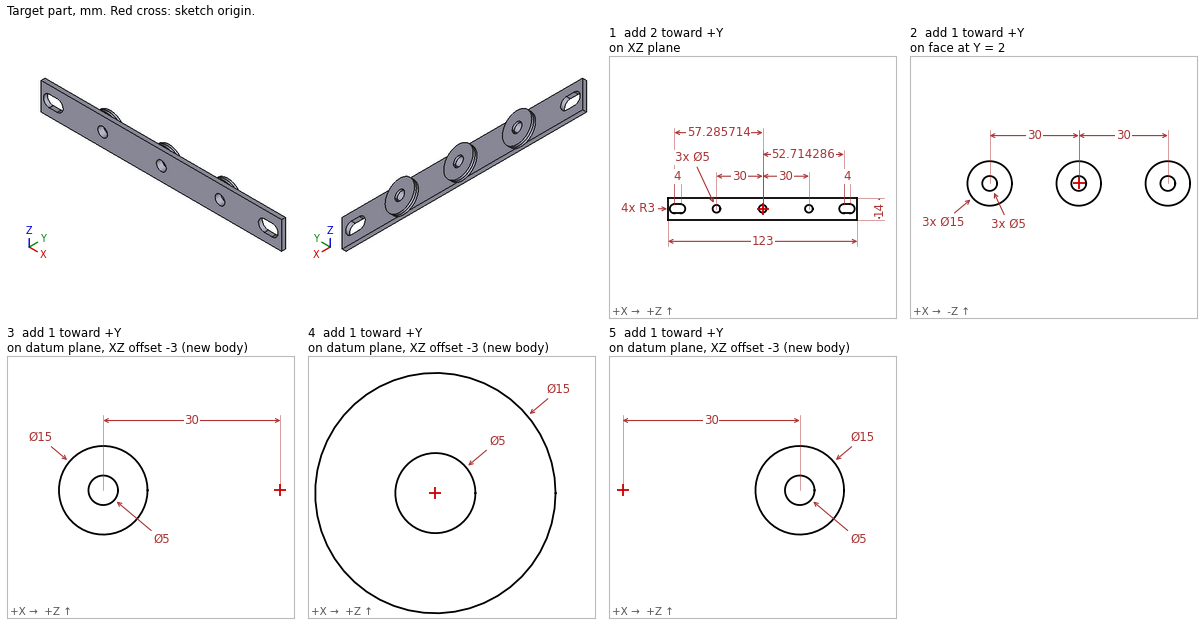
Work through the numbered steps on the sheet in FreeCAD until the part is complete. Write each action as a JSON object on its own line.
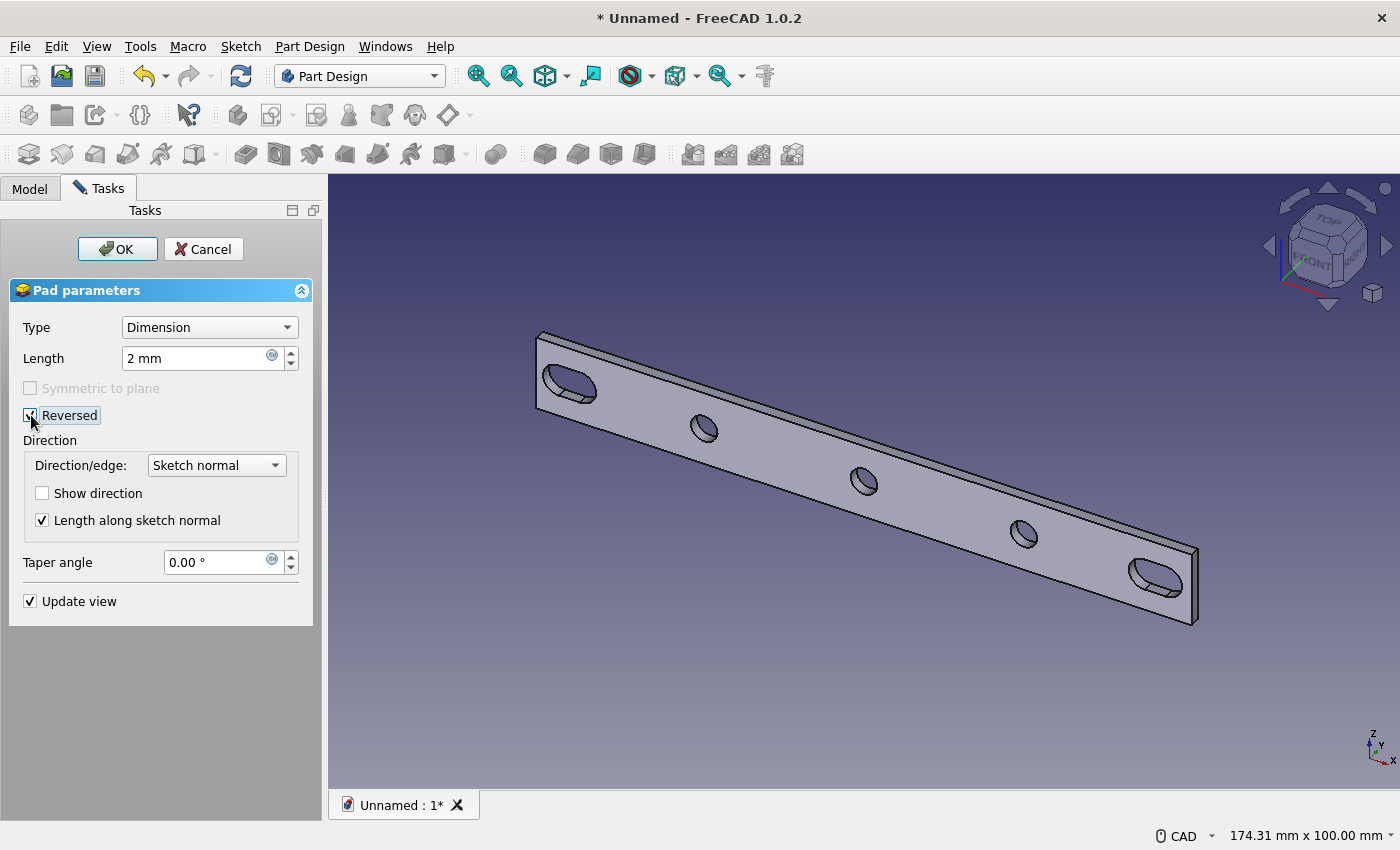
{"action": "left_click", "coordinate": [118, 249]}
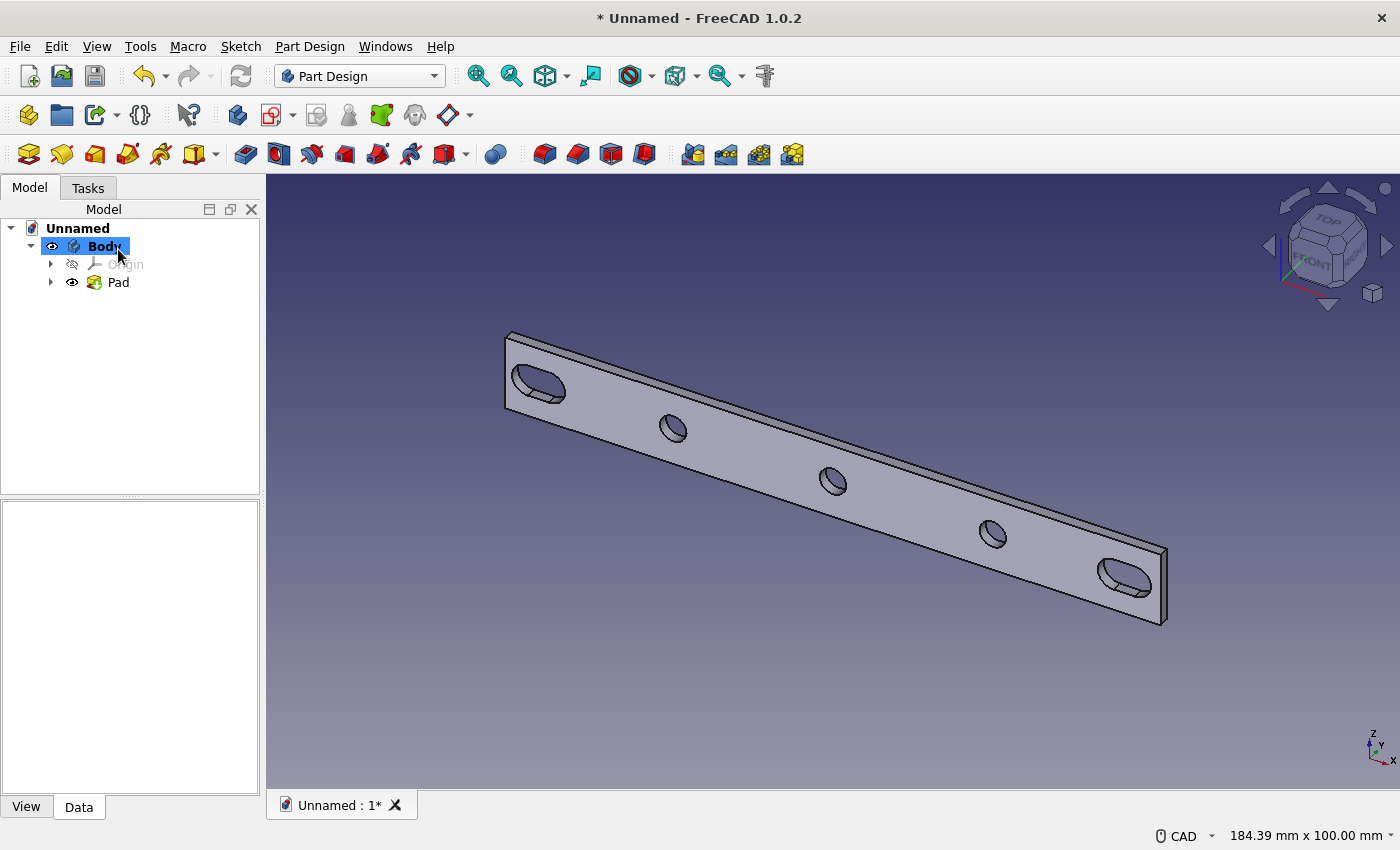
{"action": "key", "text": "4"}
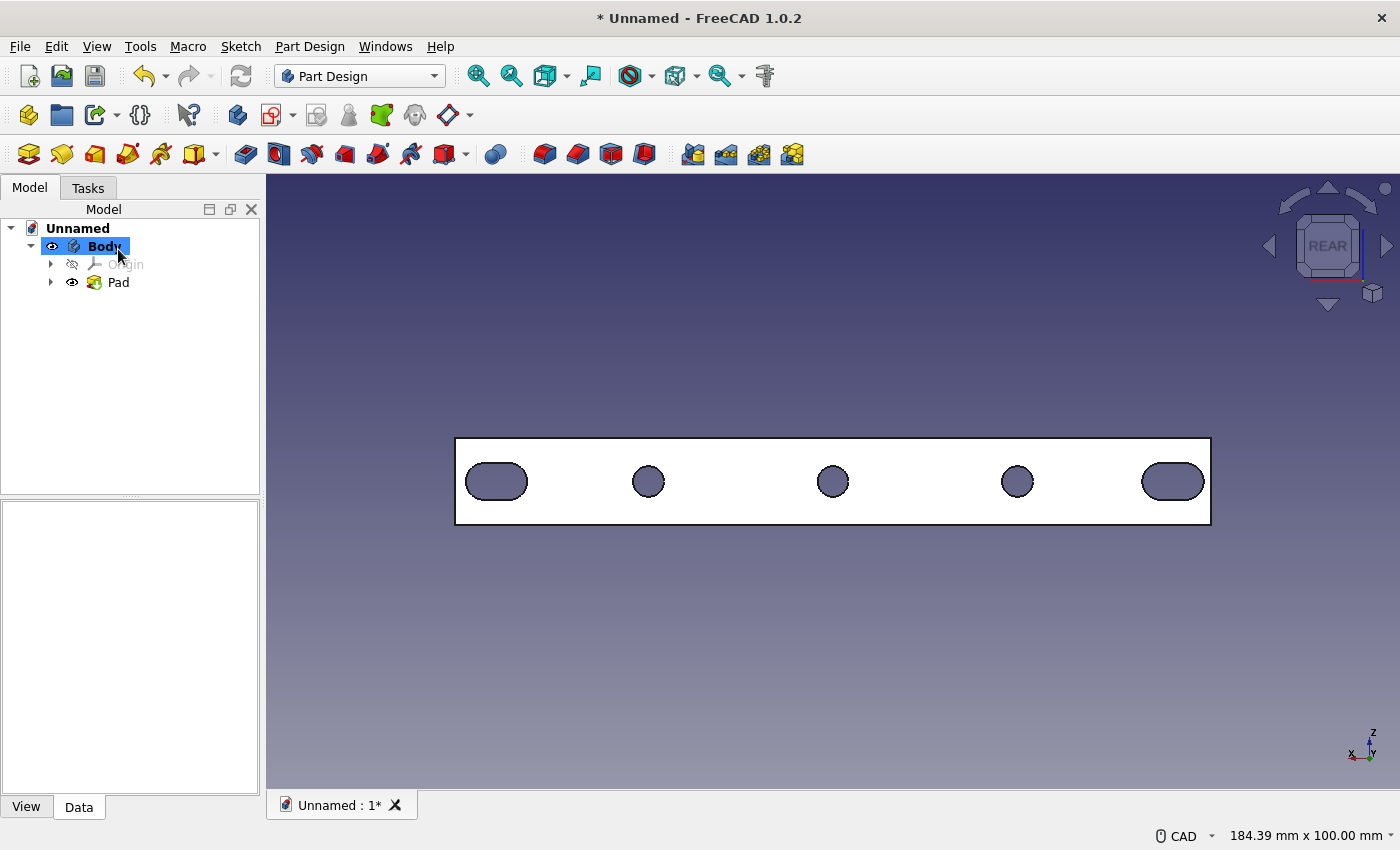
{"action": "left_click", "coordinate": [725, 480]}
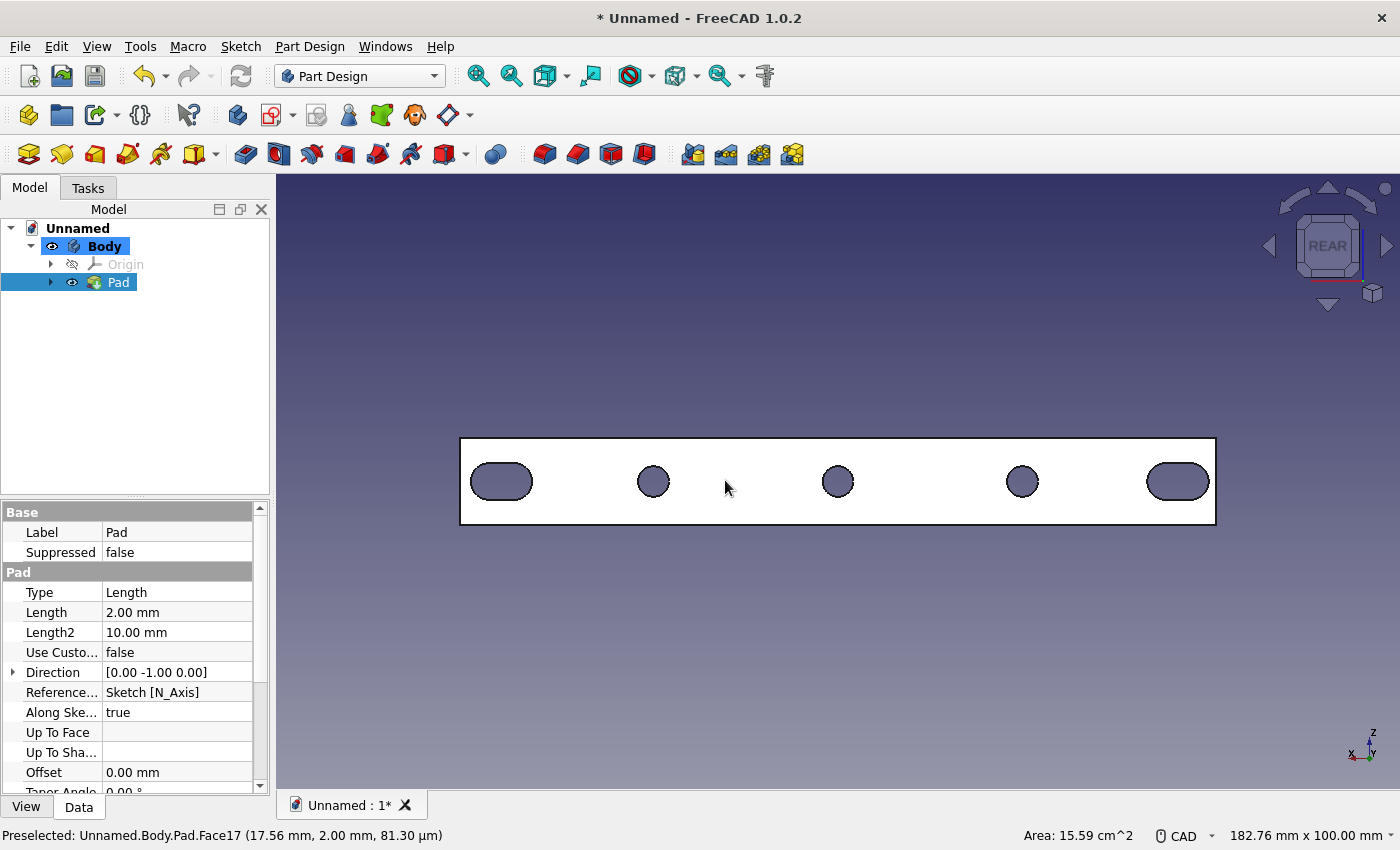
{"action": "left_click", "coordinate": [270, 116]}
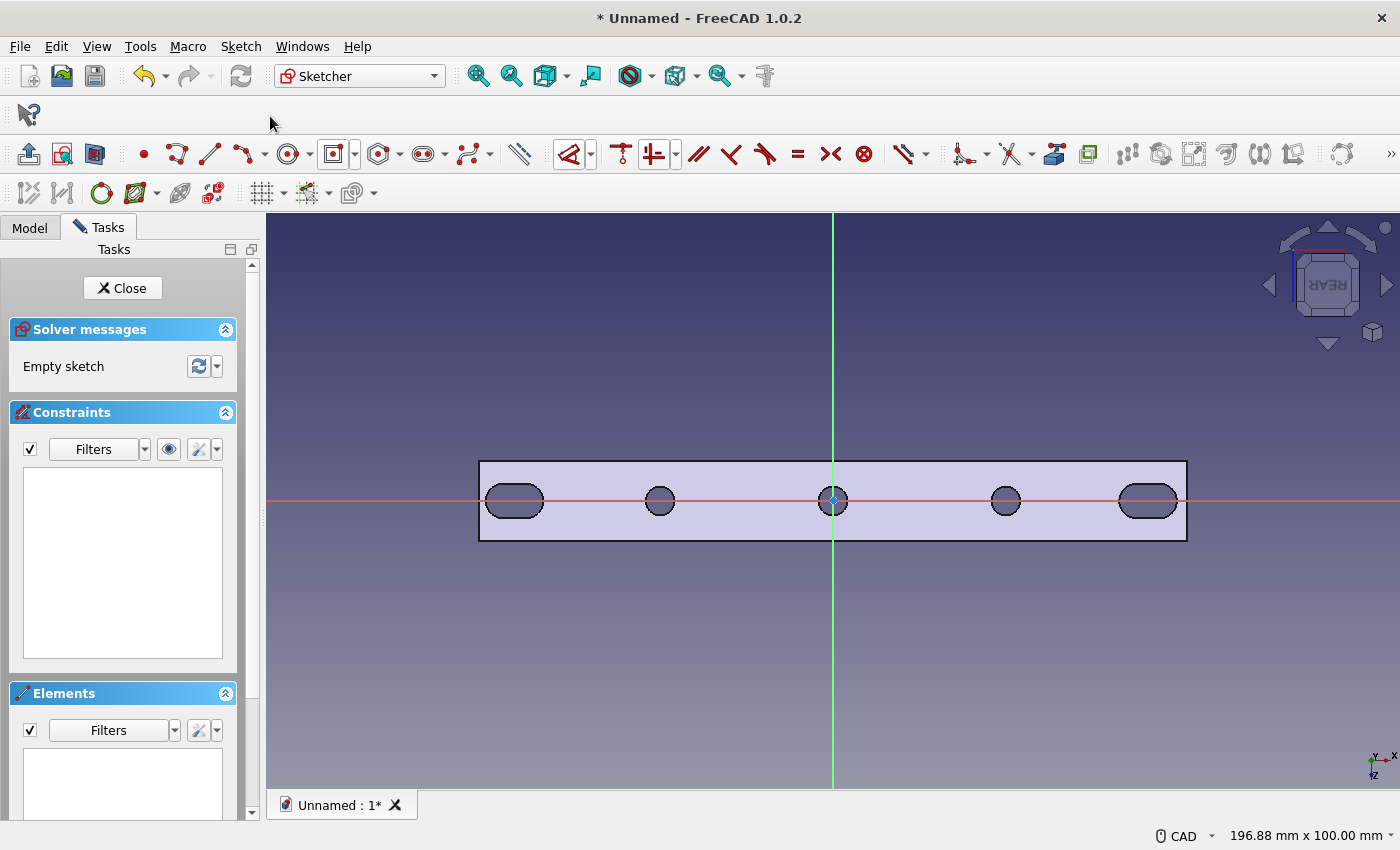
{"action": "scroll", "coordinate": [972, 501], "scroll_direction": "up", "scroll_amount": 2}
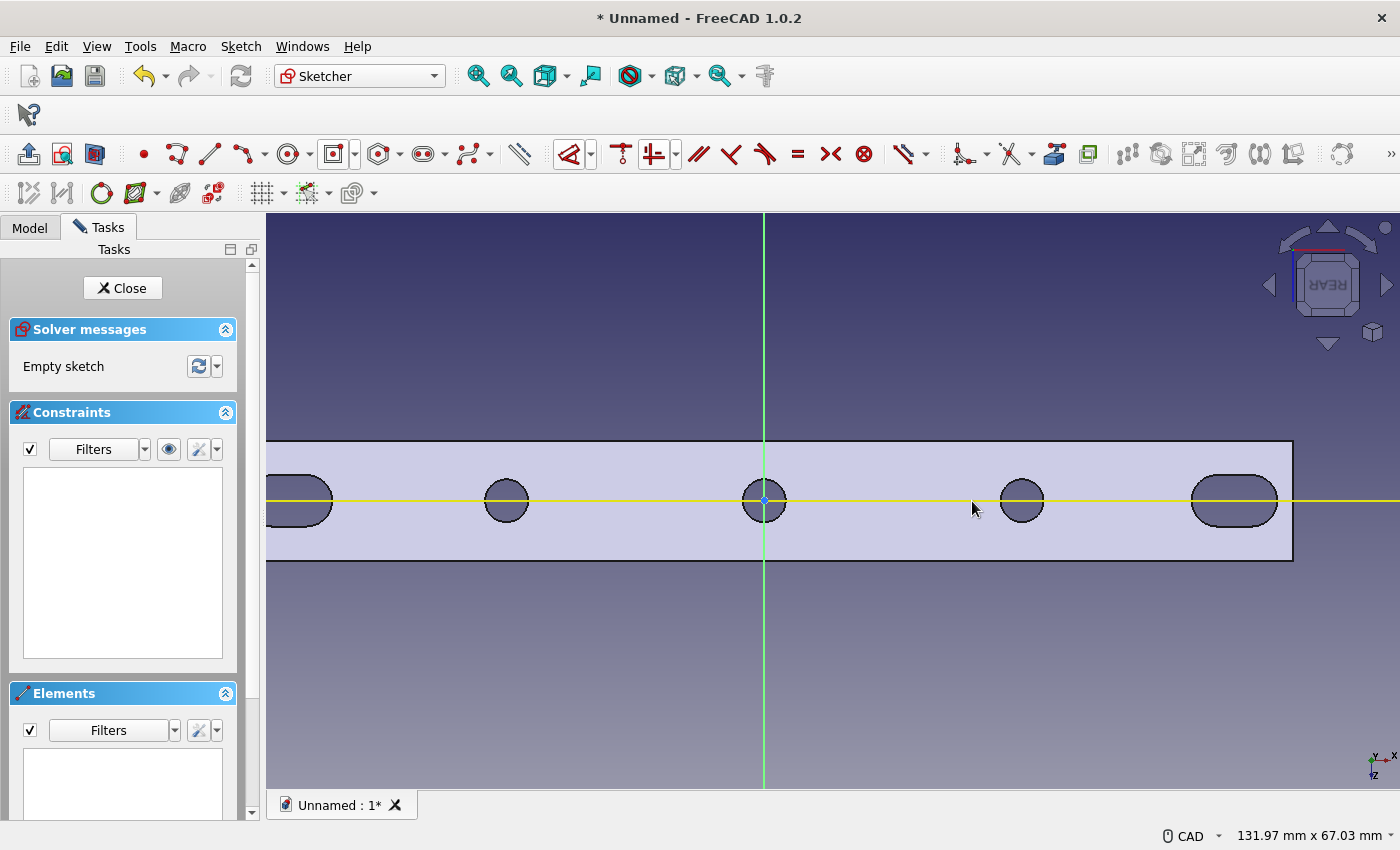
{"action": "left_click", "coordinate": [288, 154]}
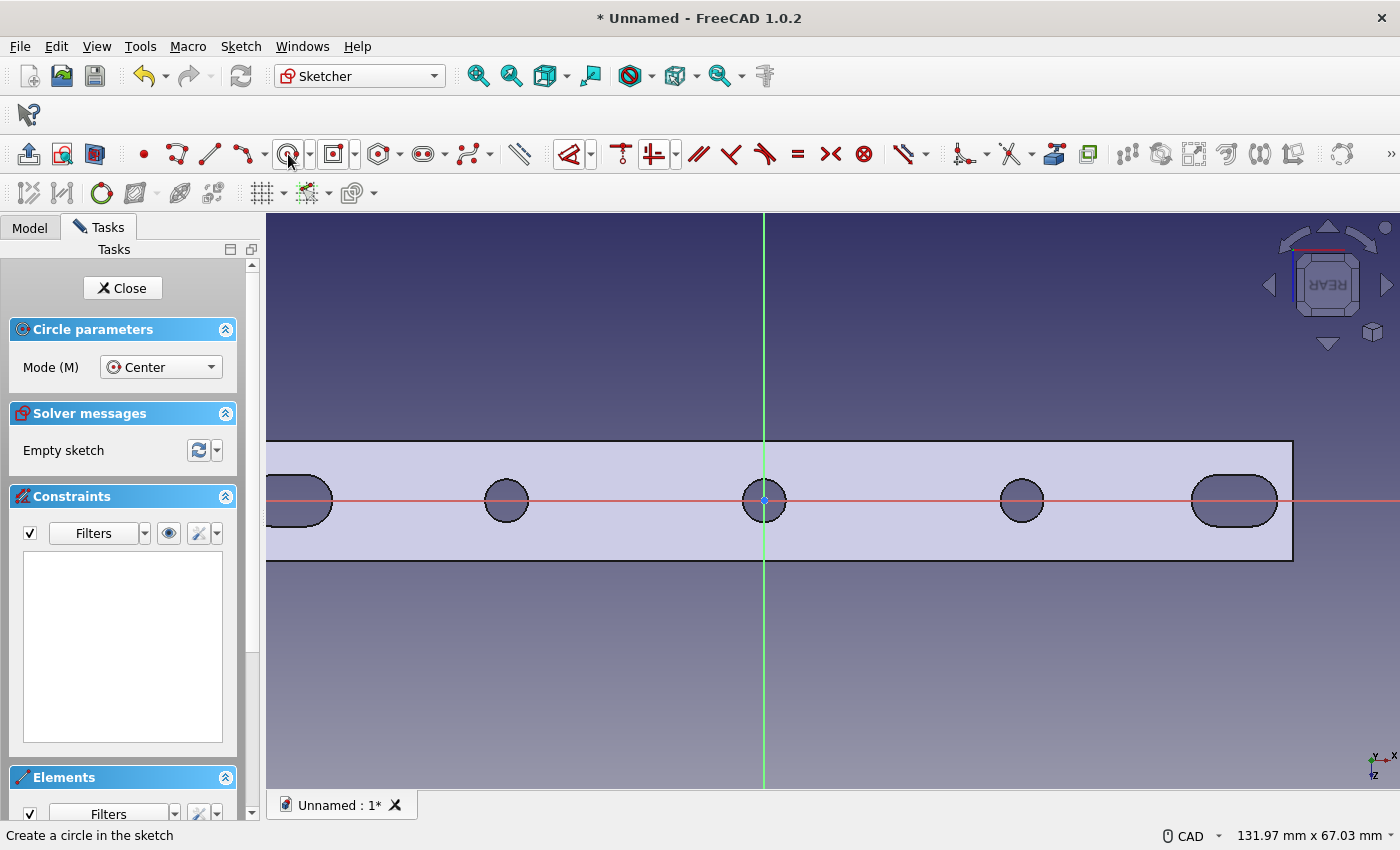
{"action": "left_click", "coordinate": [507, 501]}
{"action": "left_click", "coordinate": [552, 455]}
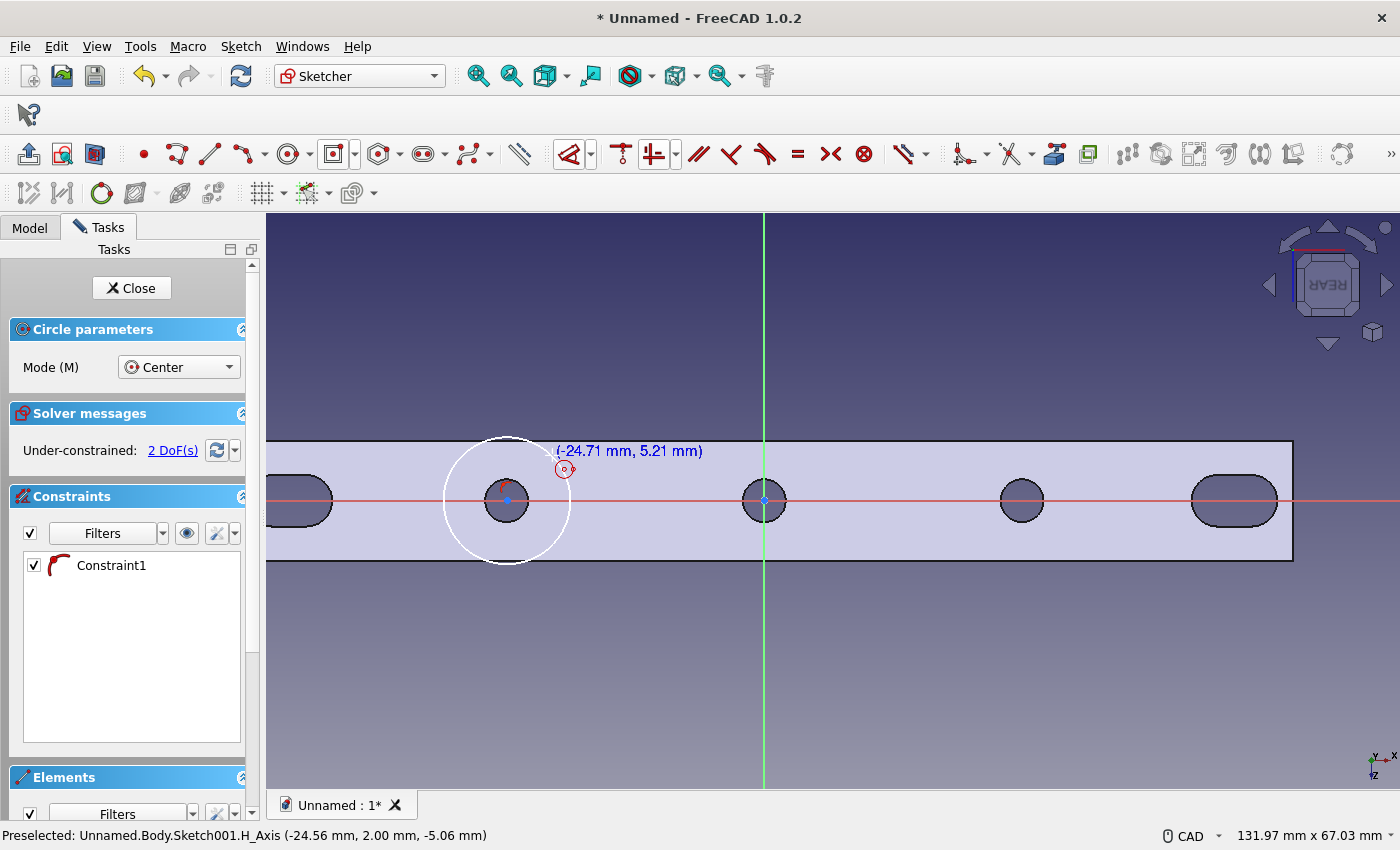
{"action": "left_click", "coordinate": [764, 501]}
{"action": "left_click", "coordinate": [810, 455]}